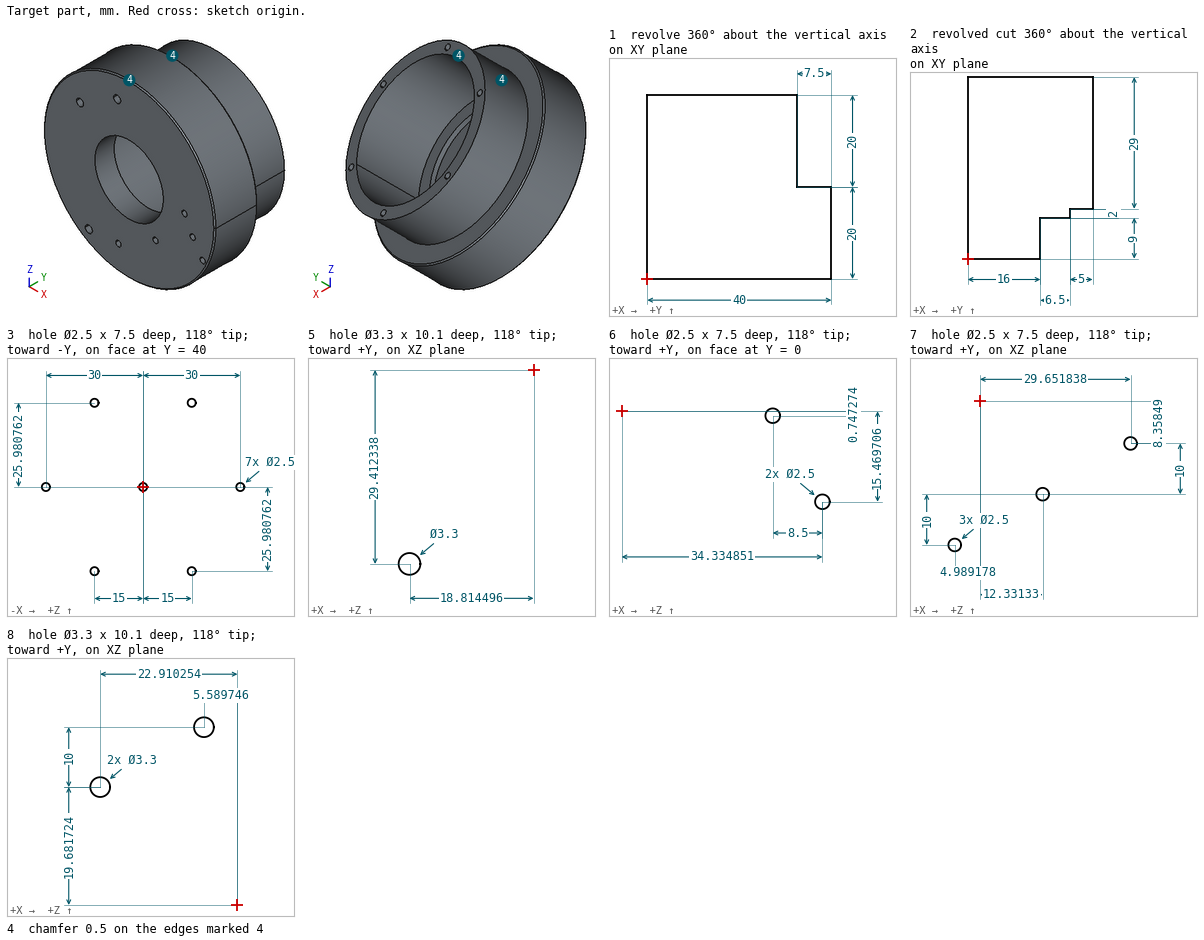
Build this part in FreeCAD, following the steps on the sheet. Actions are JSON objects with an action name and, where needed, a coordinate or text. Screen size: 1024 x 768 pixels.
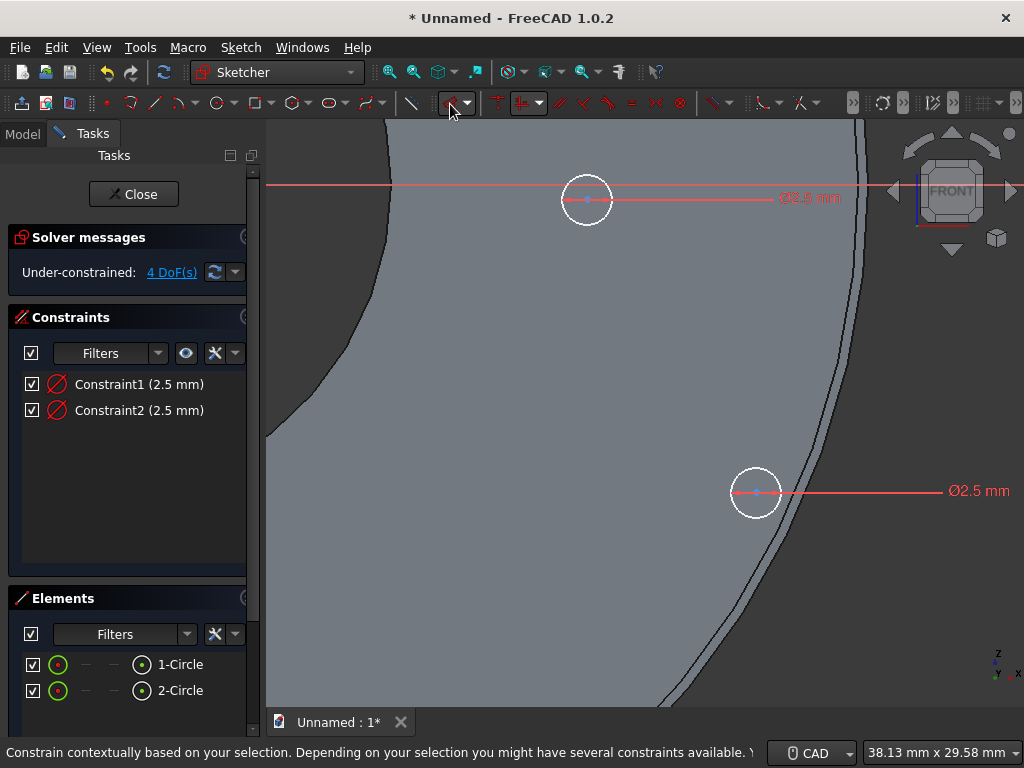
{"action": "left_click", "coordinate": [756, 493]}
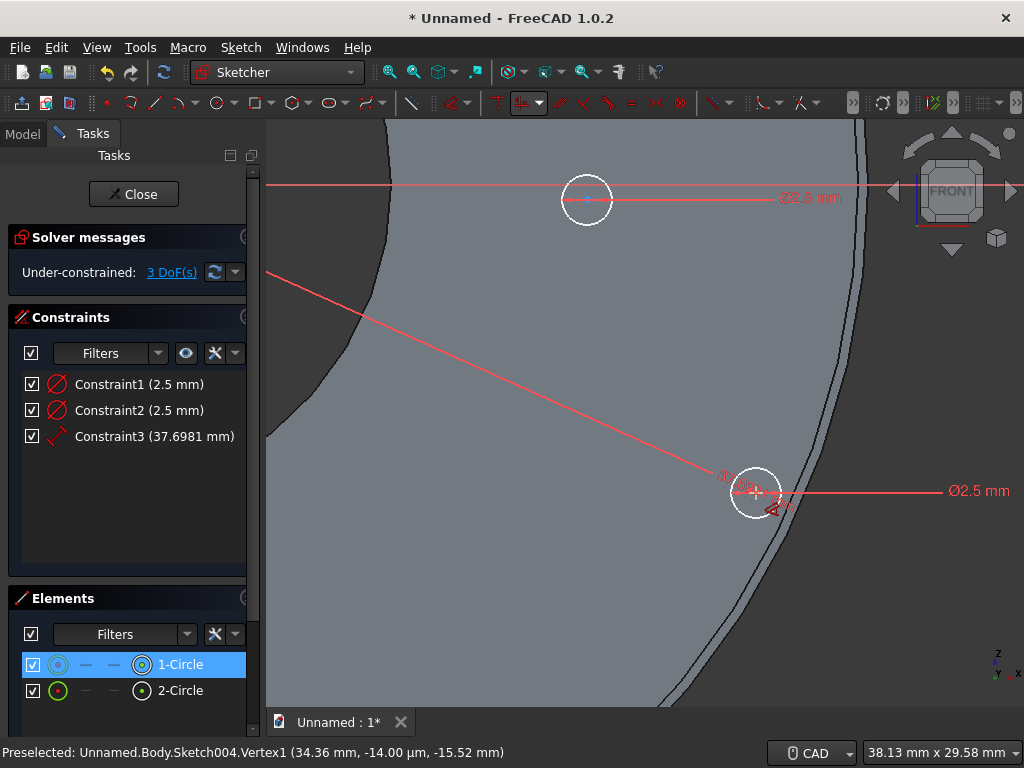
{"action": "left_click", "coordinate": [587, 200]}
{"action": "left_click", "coordinate": [672, 527]}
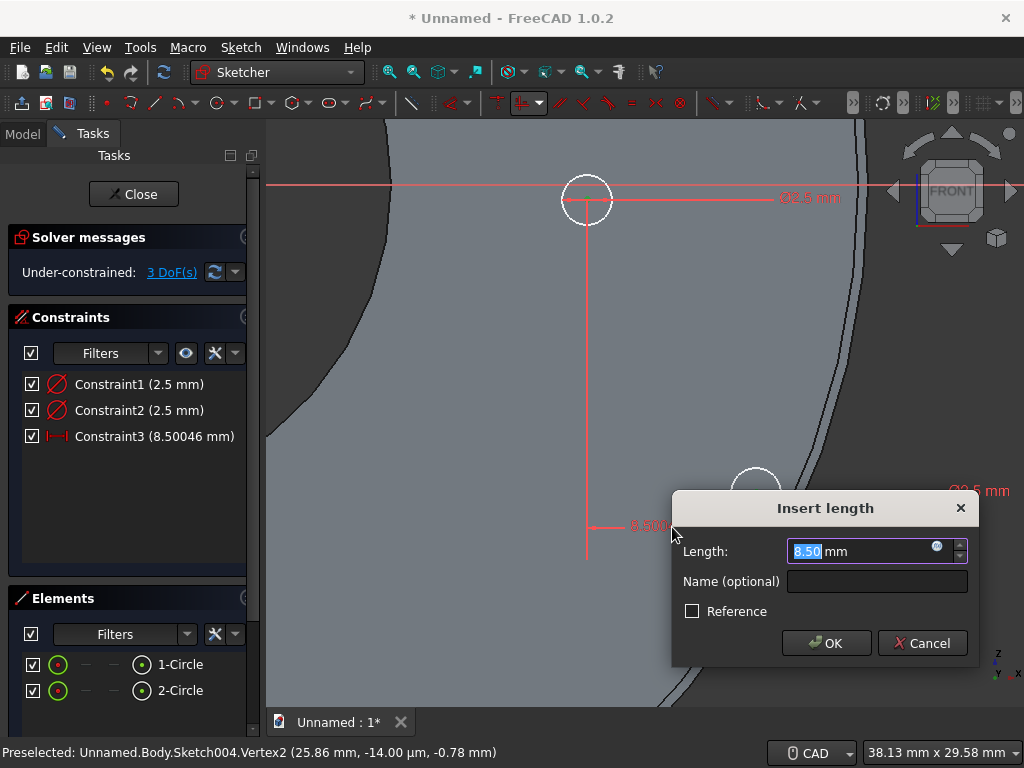
{"action": "type", "text": "8.5"}
{"action": "key", "text": "Return"}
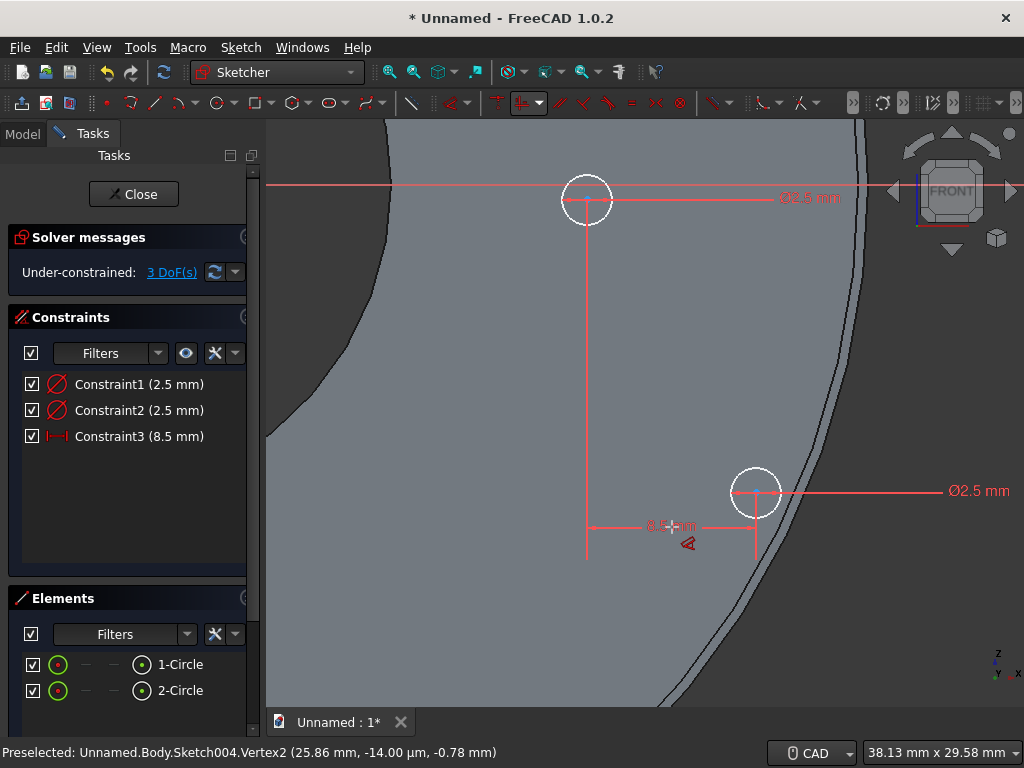
{"action": "scroll", "coordinate": [587, 200], "scroll_direction": "up", "scroll_amount": 5}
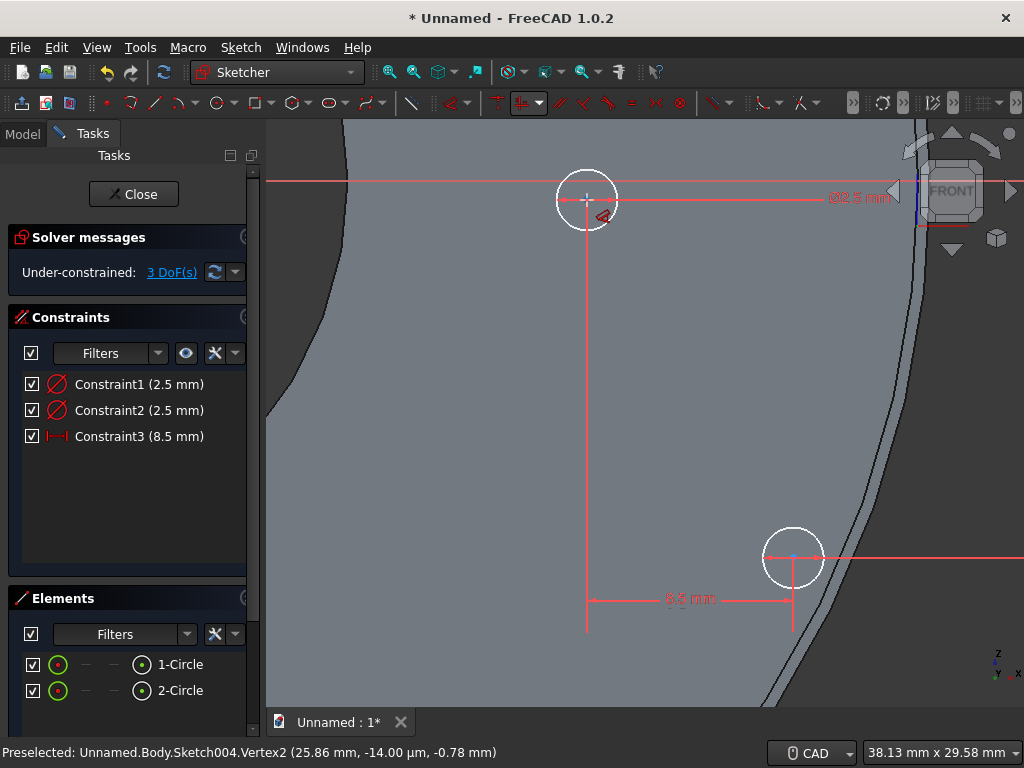
{"action": "left_click", "coordinate": [586, 200]}
{"action": "left_click", "coordinate": [620, 179]}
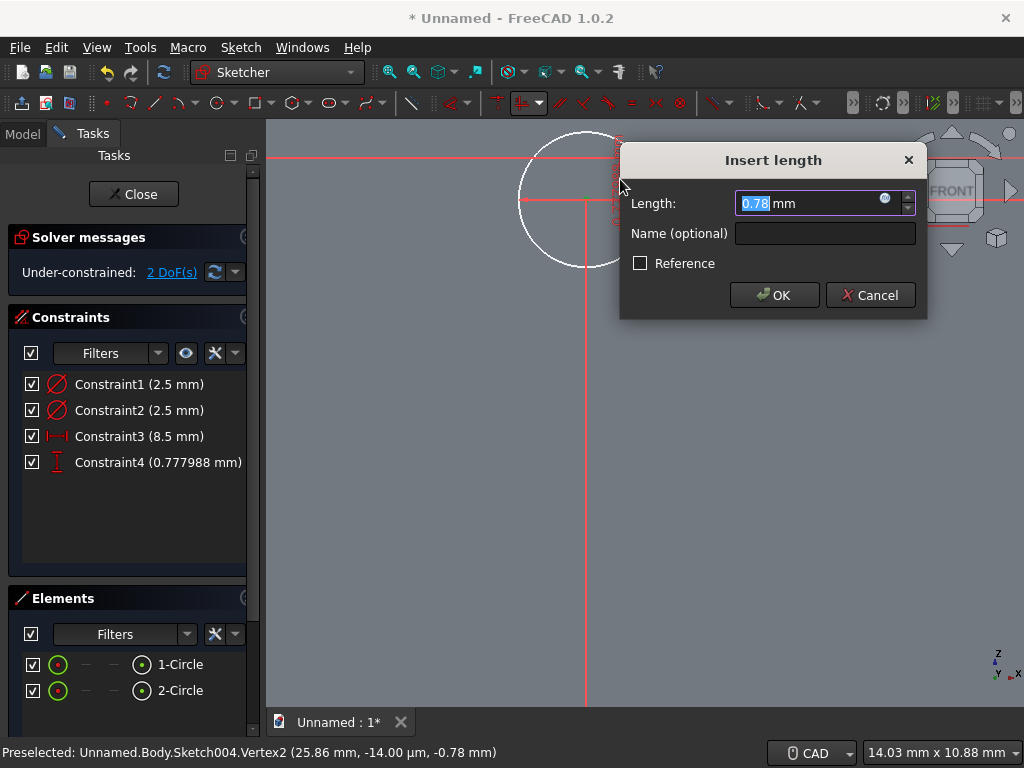
{"action": "type", "text": "0.747274"}
{"action": "key", "text": "Return"}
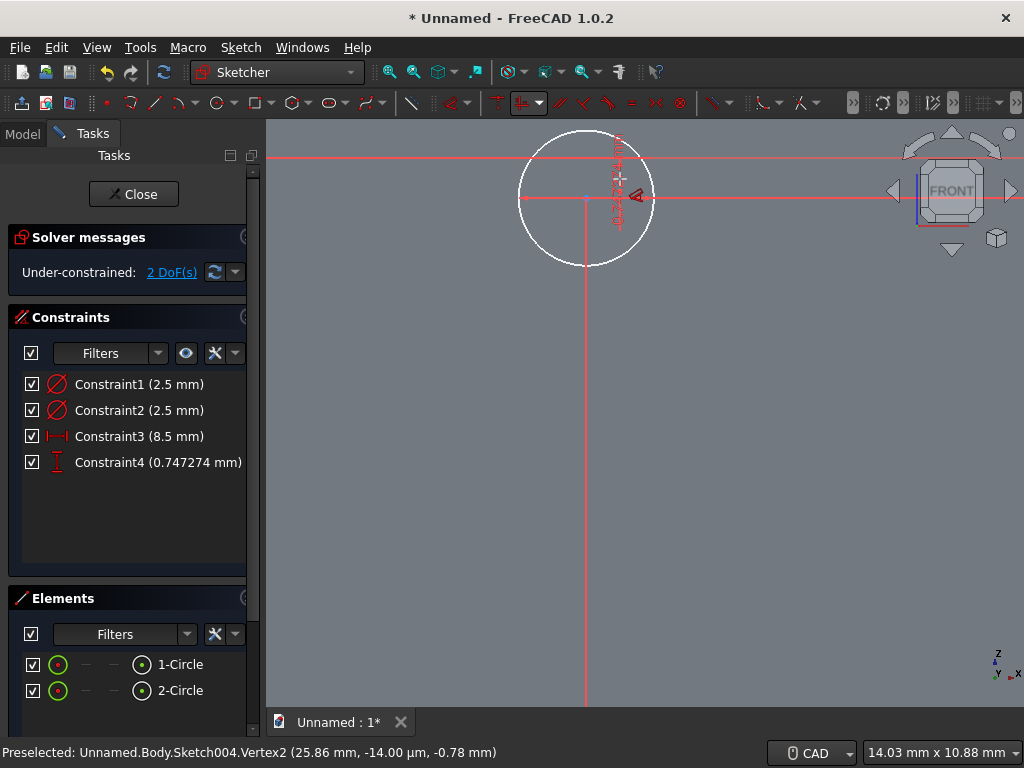
{"action": "scroll", "coordinate": [684, 367], "scroll_direction": "down", "scroll_amount": 8}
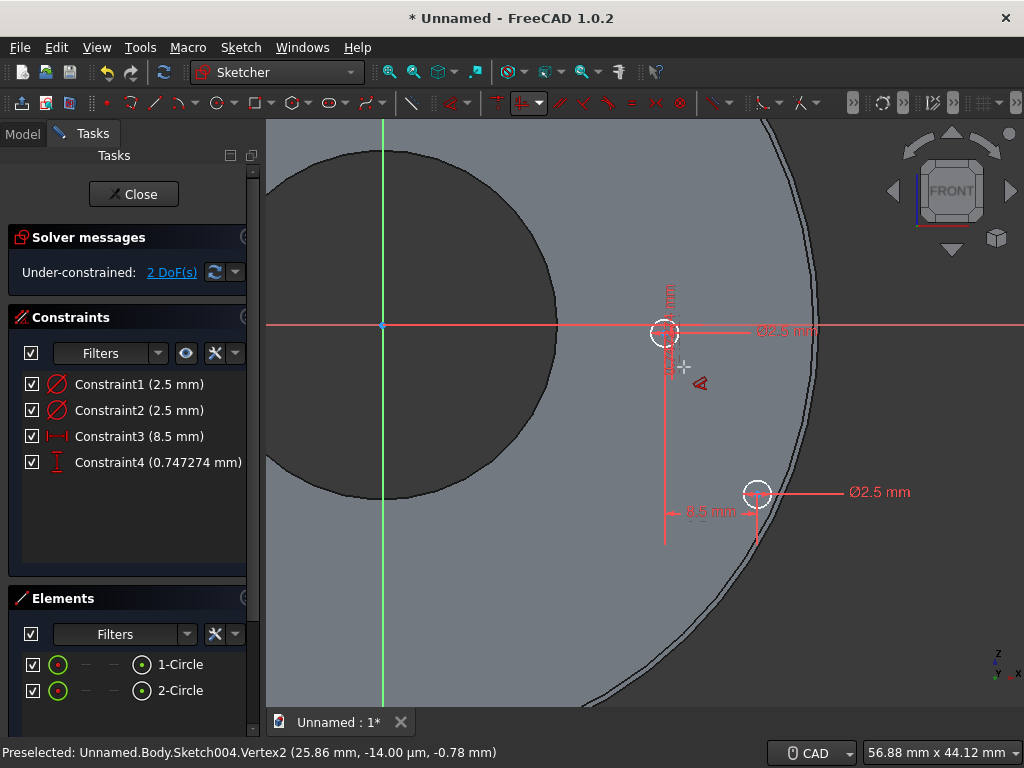
{"action": "left_click", "coordinate": [757, 494]}
{"action": "left_click", "coordinate": [570, 291]}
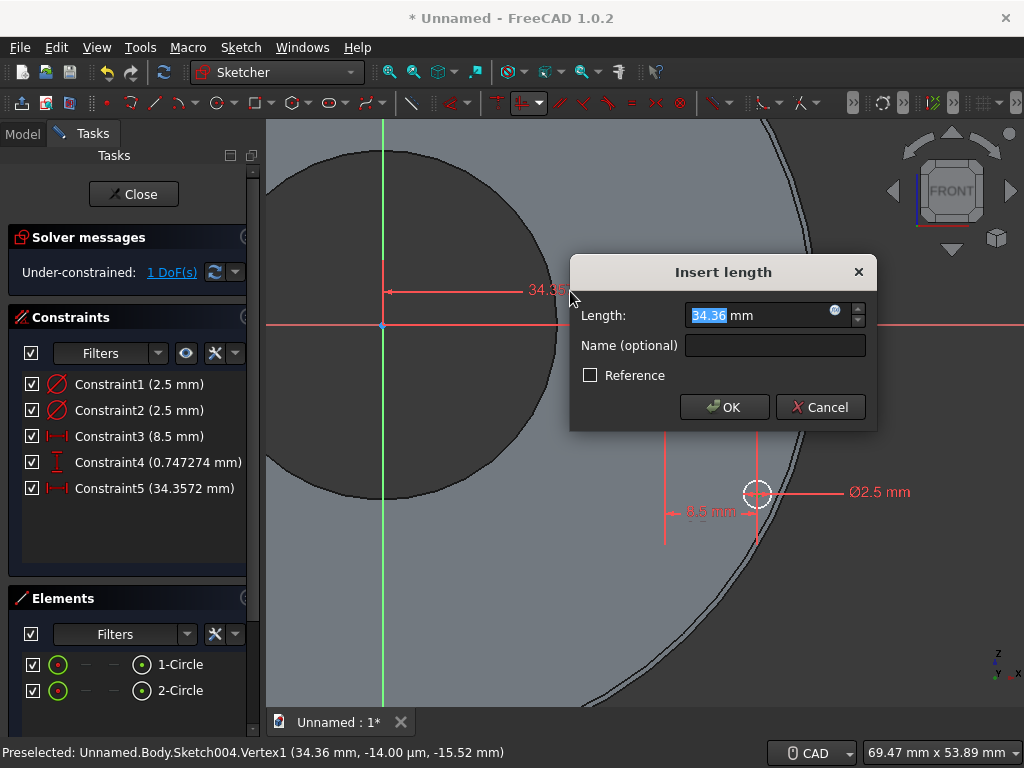
{"action": "type", "text": "34.334851"}
{"action": "key", "text": "Return"}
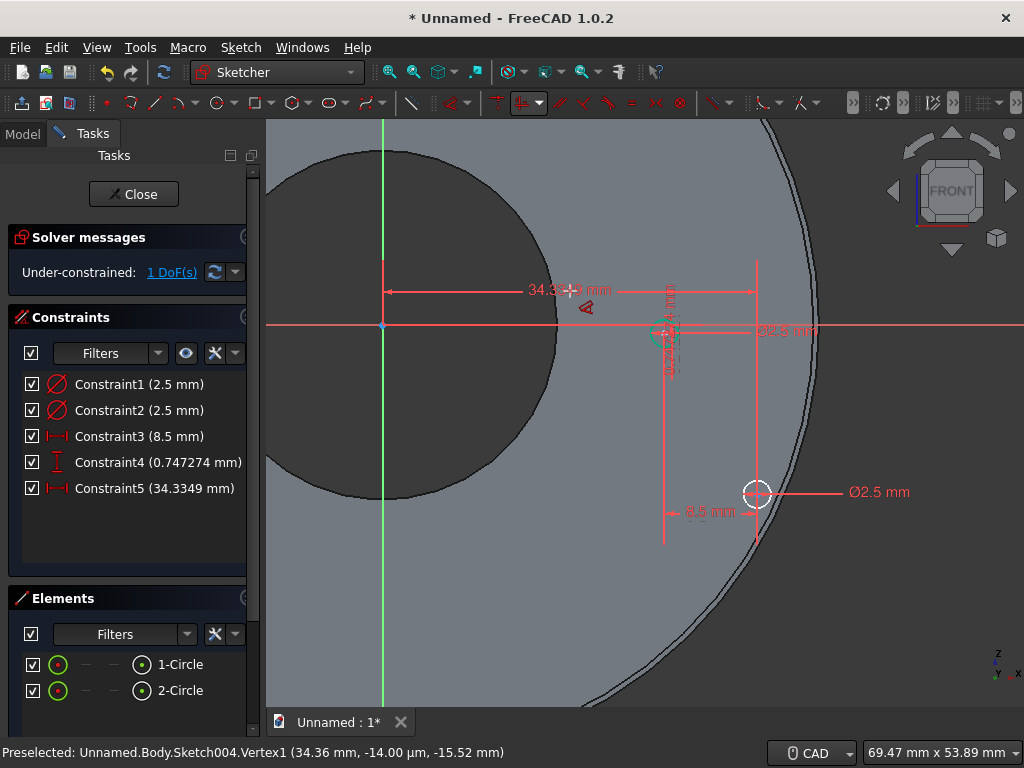
{"action": "left_click", "coordinate": [757, 494]}
{"action": "left_click", "coordinate": [349, 410]}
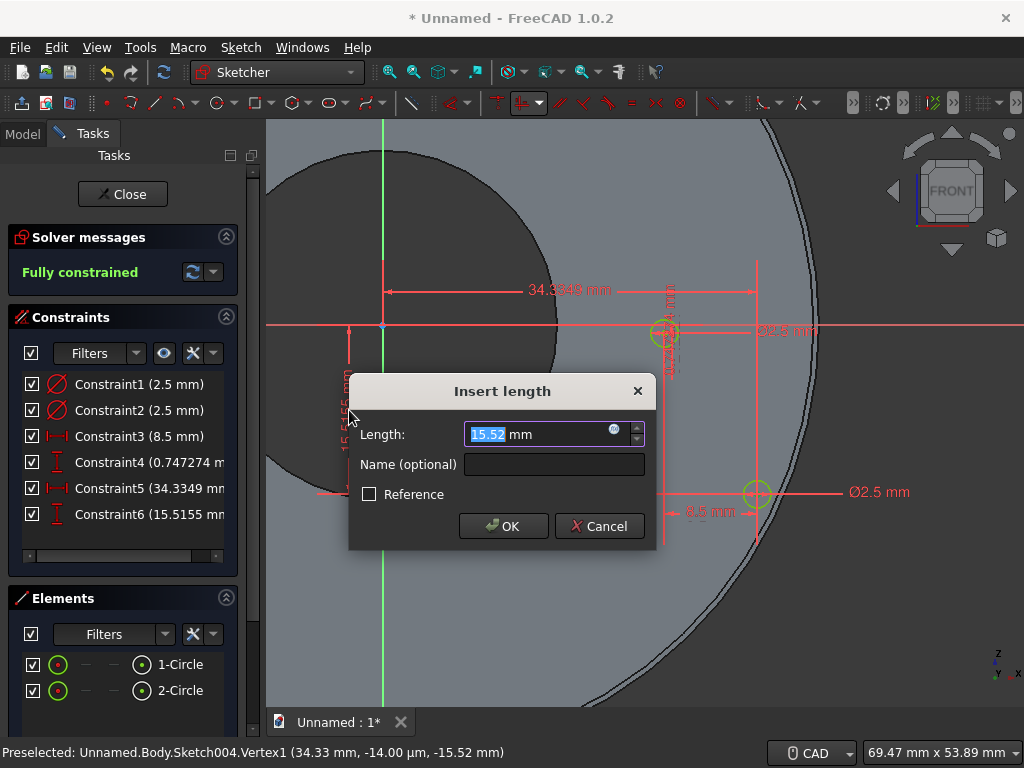
{"action": "type", "text": "15.469706"}
{"action": "key", "text": "Return"}
{"action": "key", "text": "Escape"}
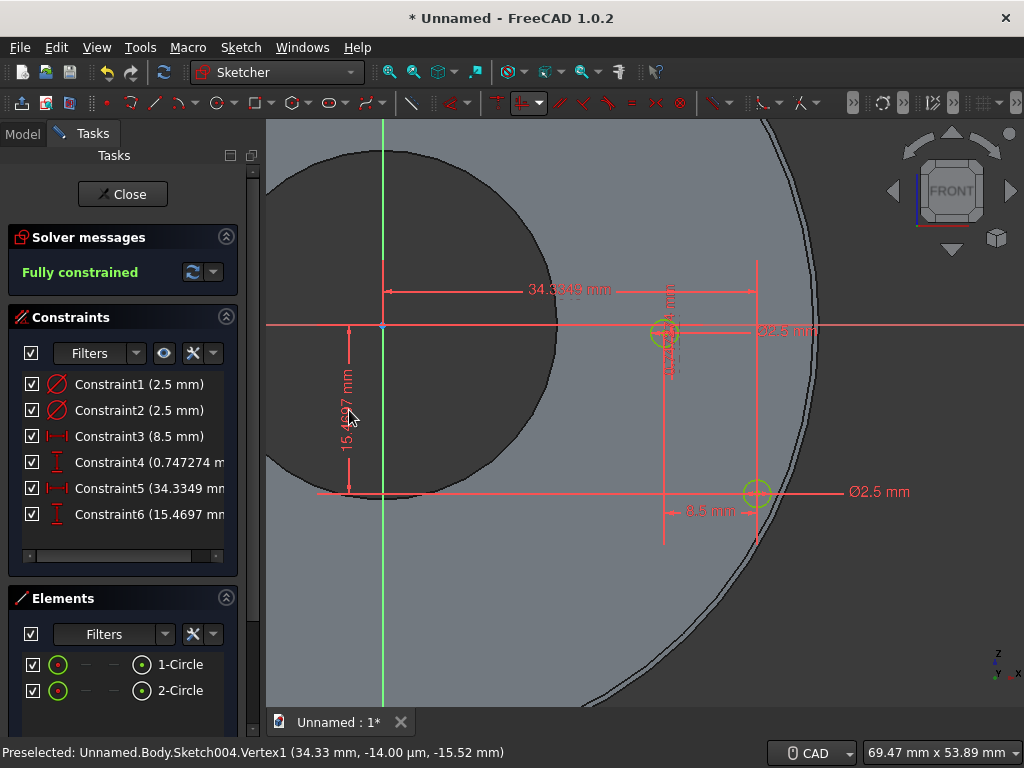
{"action": "left_click", "coordinate": [123, 194]}